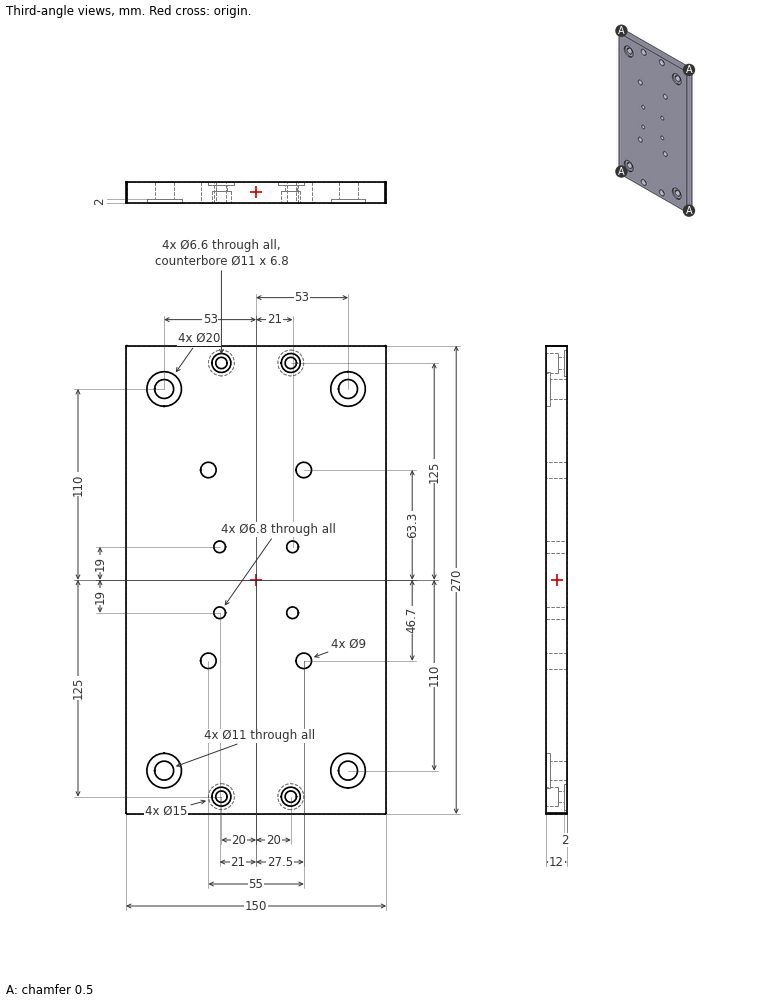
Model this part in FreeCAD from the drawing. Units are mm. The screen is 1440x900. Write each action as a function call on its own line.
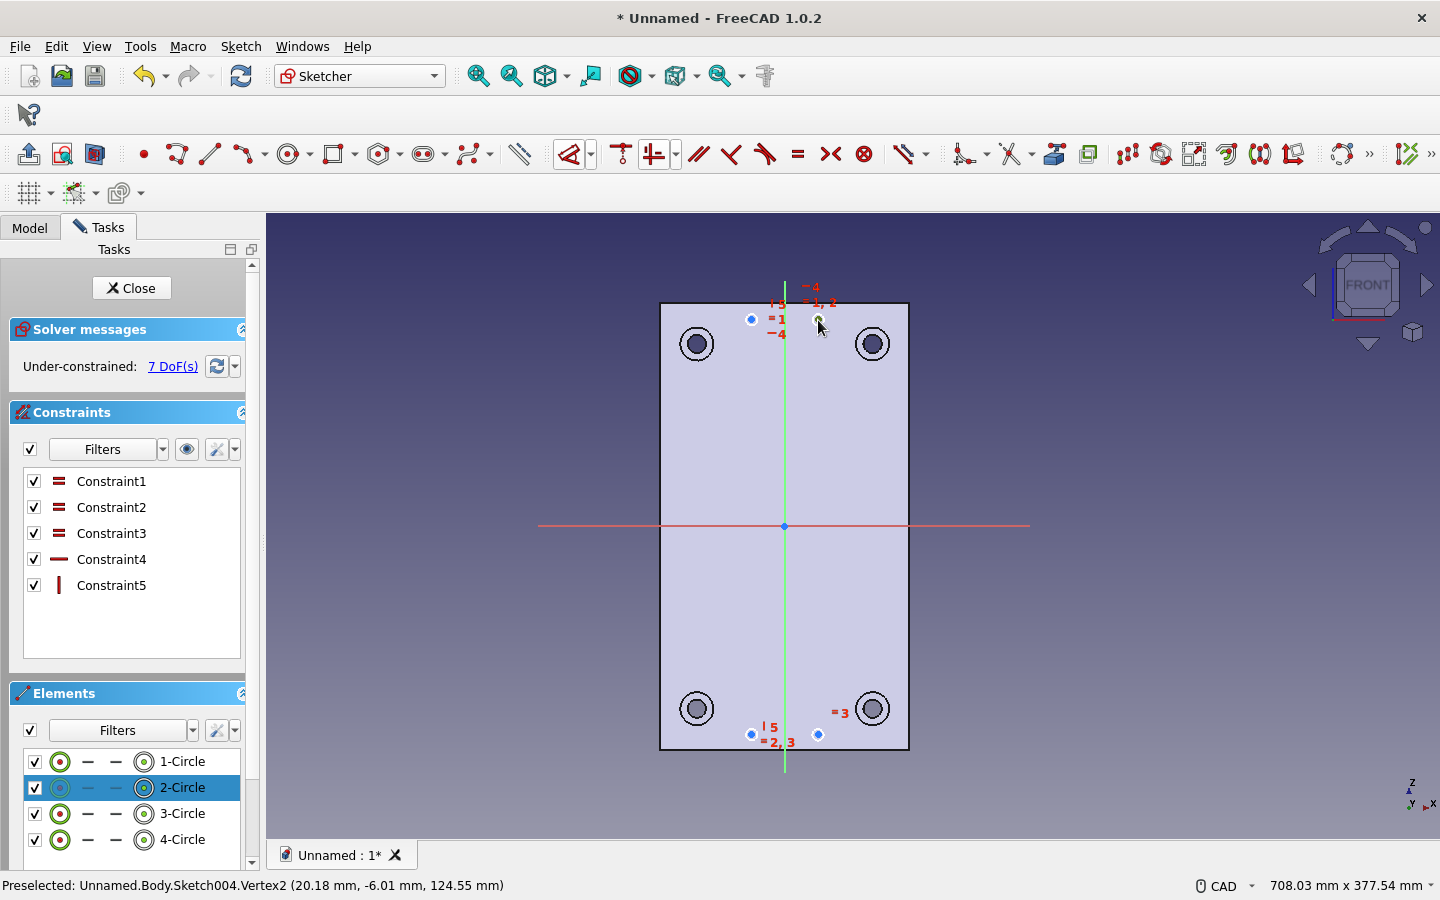
click(818, 735)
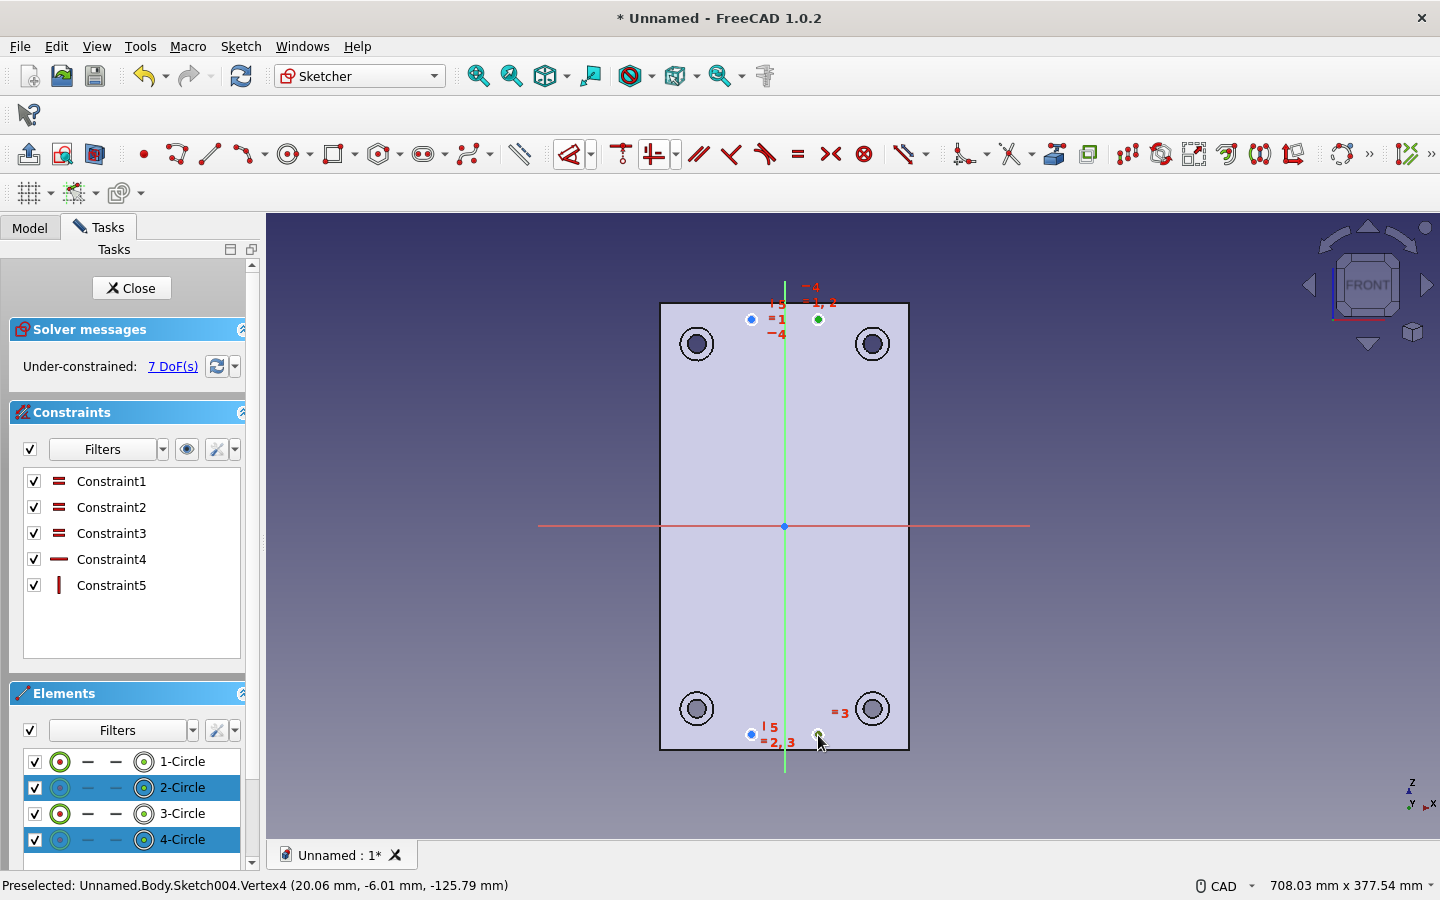
key(v)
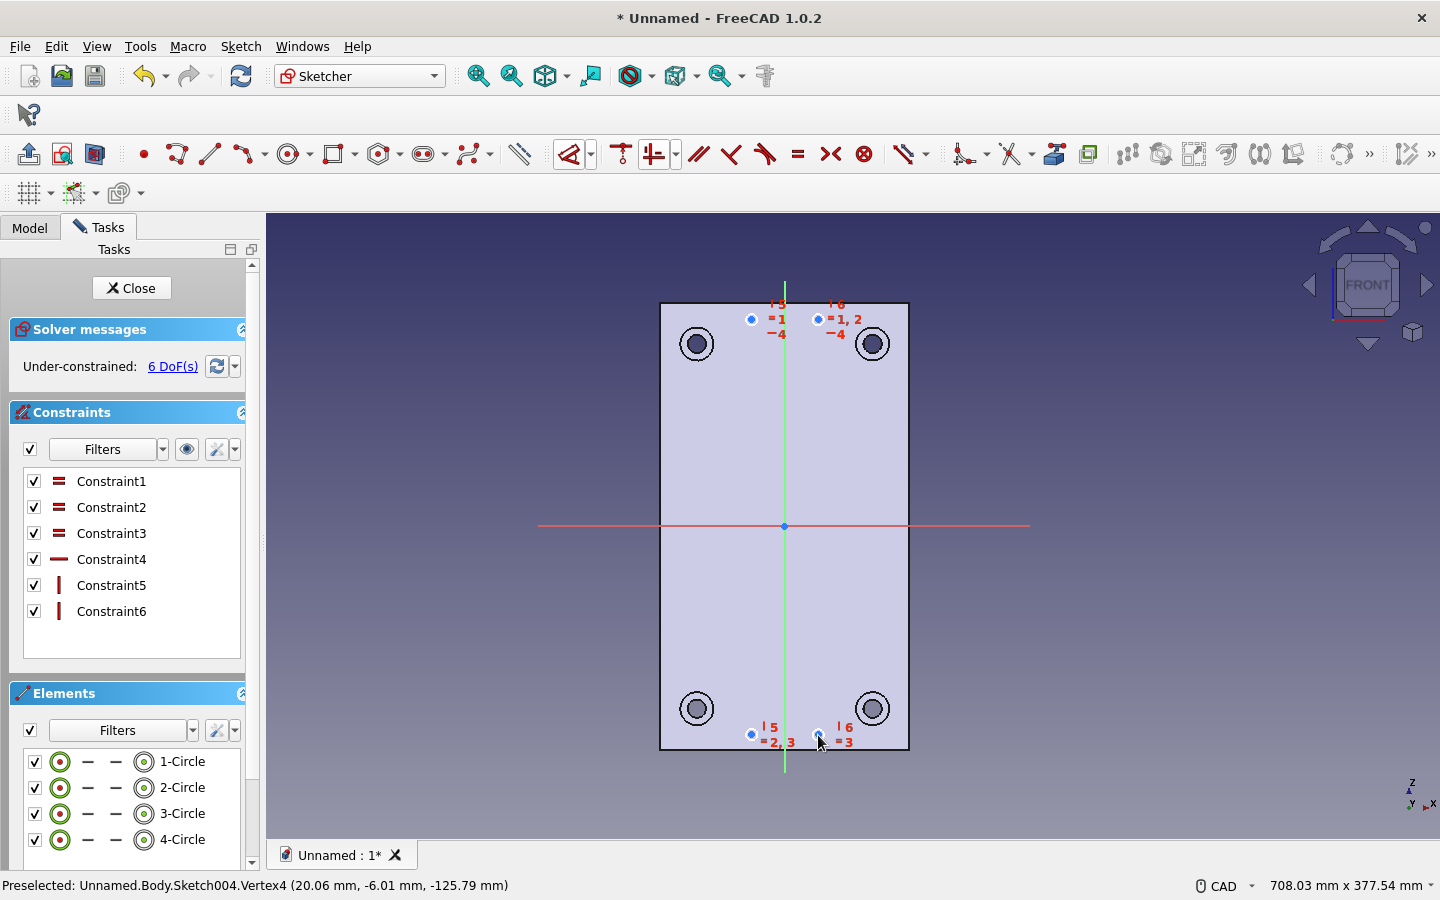
click(752, 735)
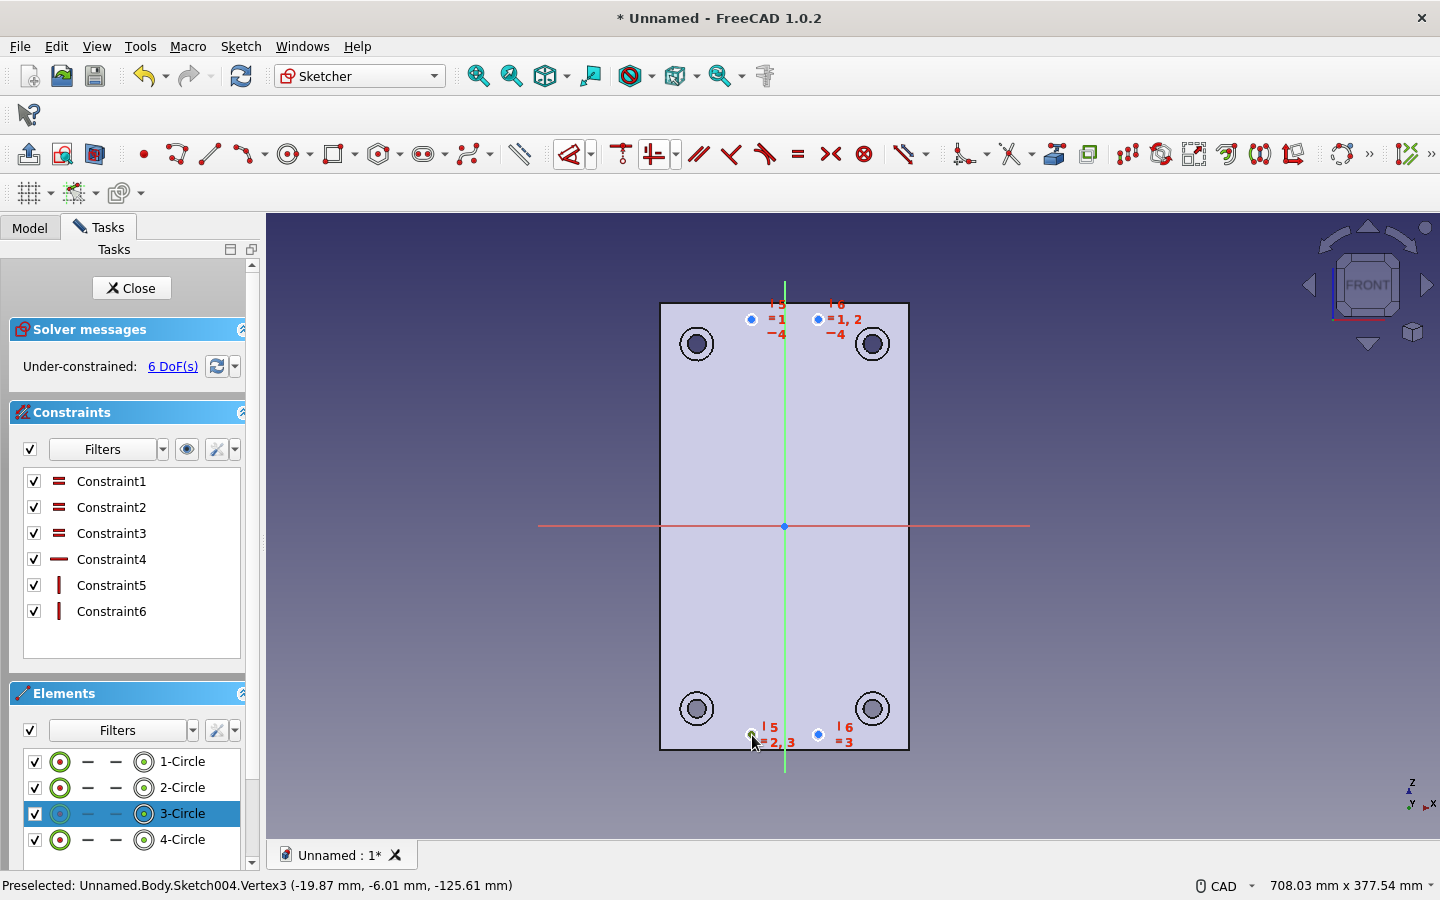
click(818, 735)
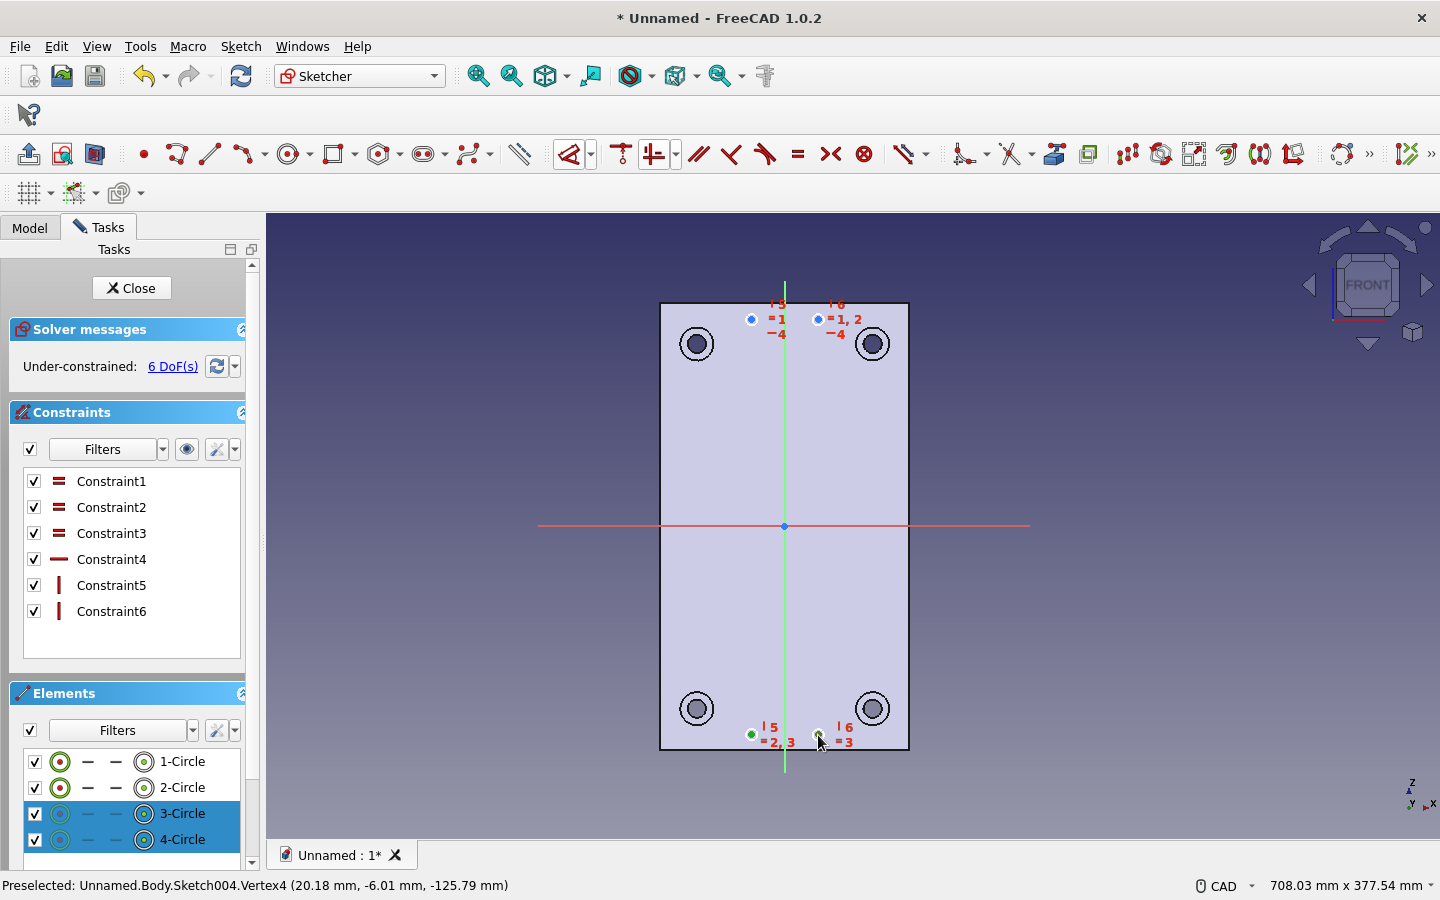
click(676, 154)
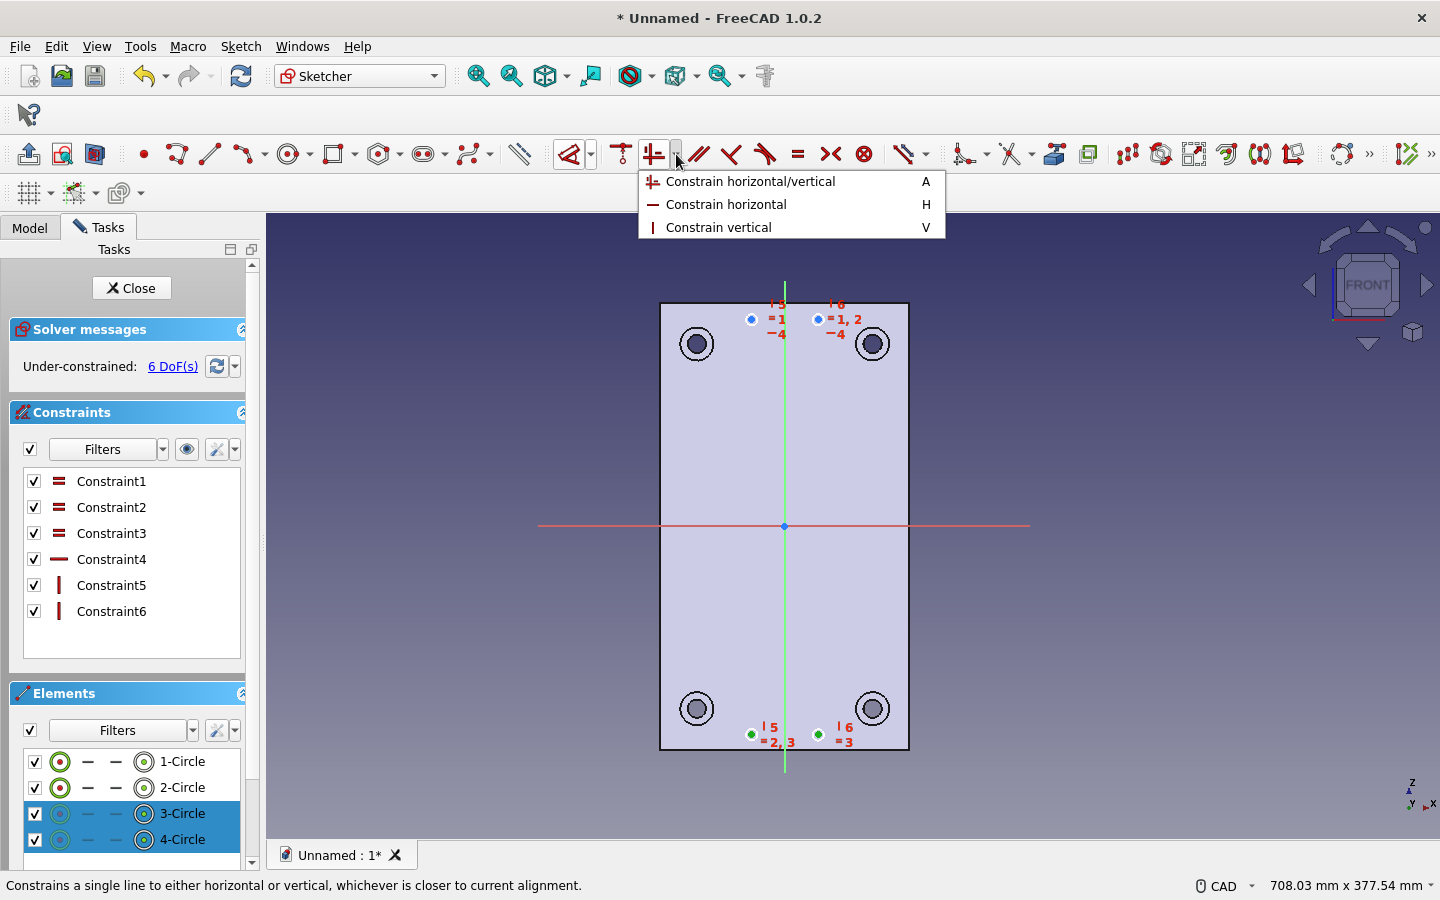
click(792, 204)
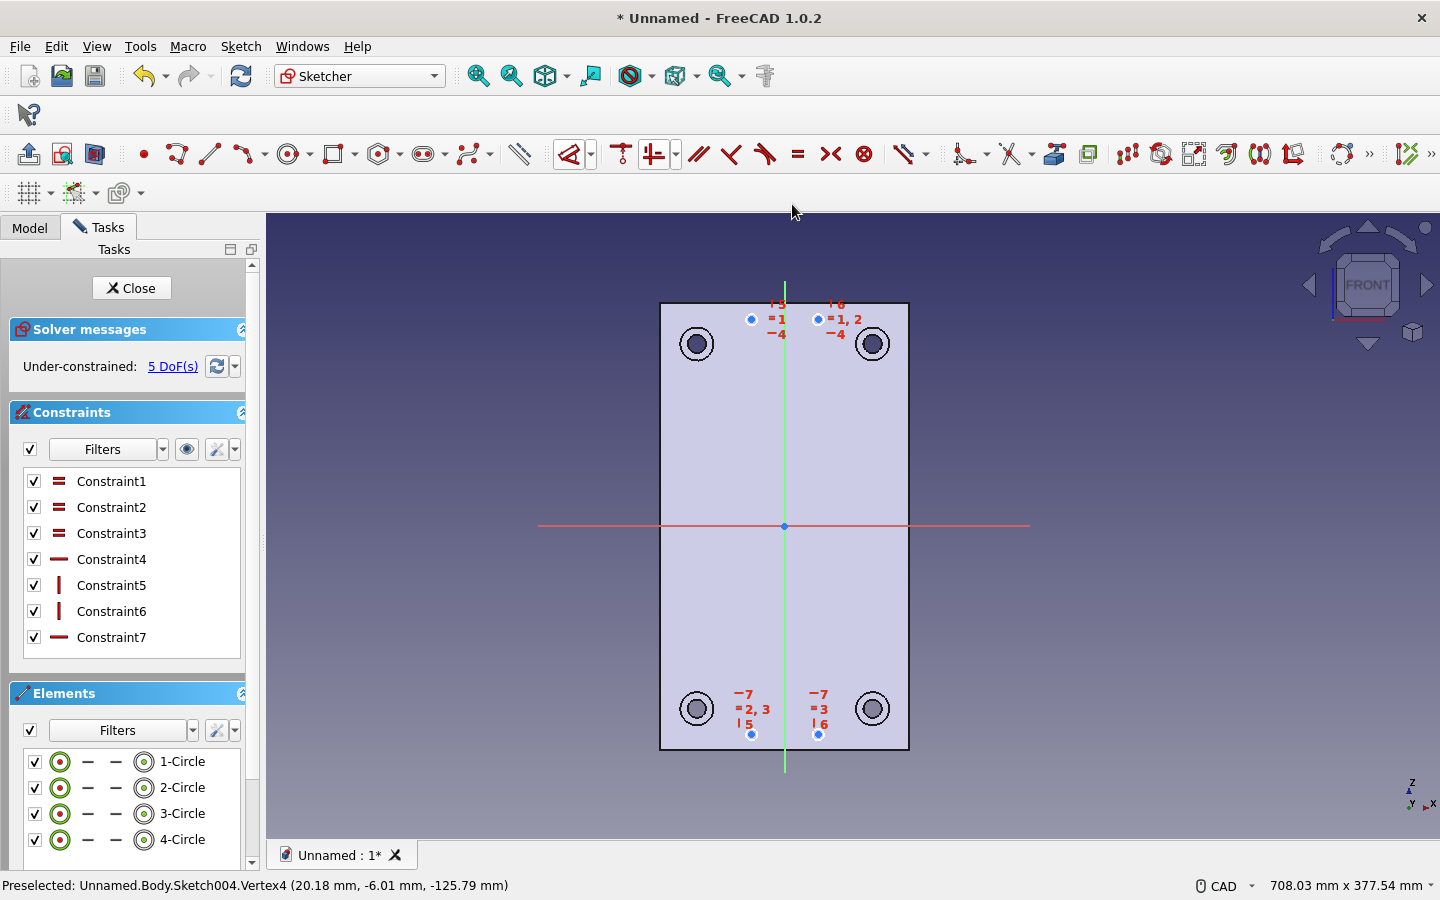
scroll(757, 320, up, 7)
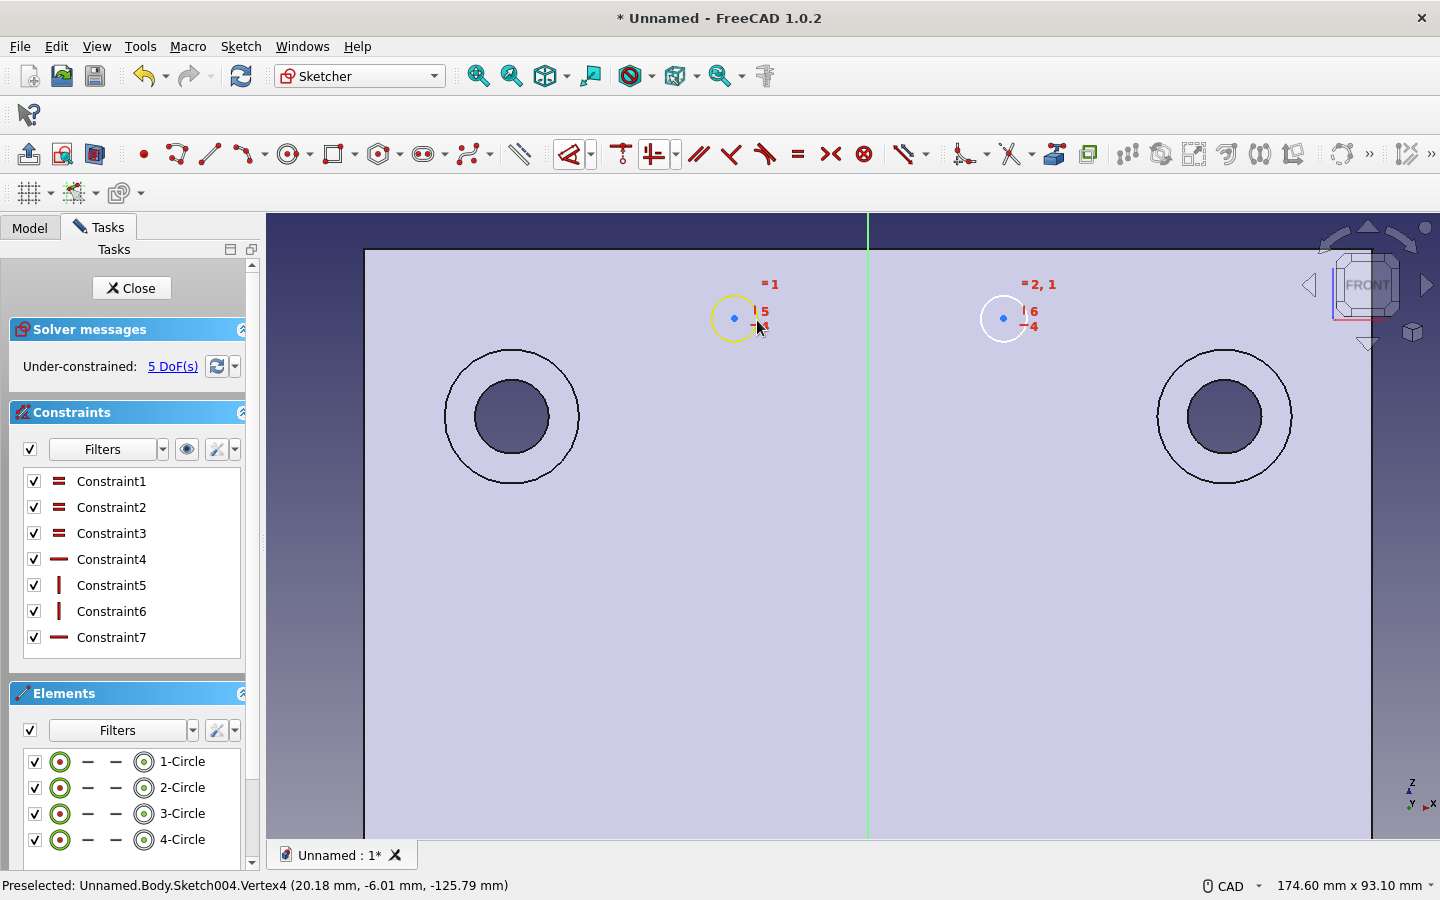
click(712, 318)